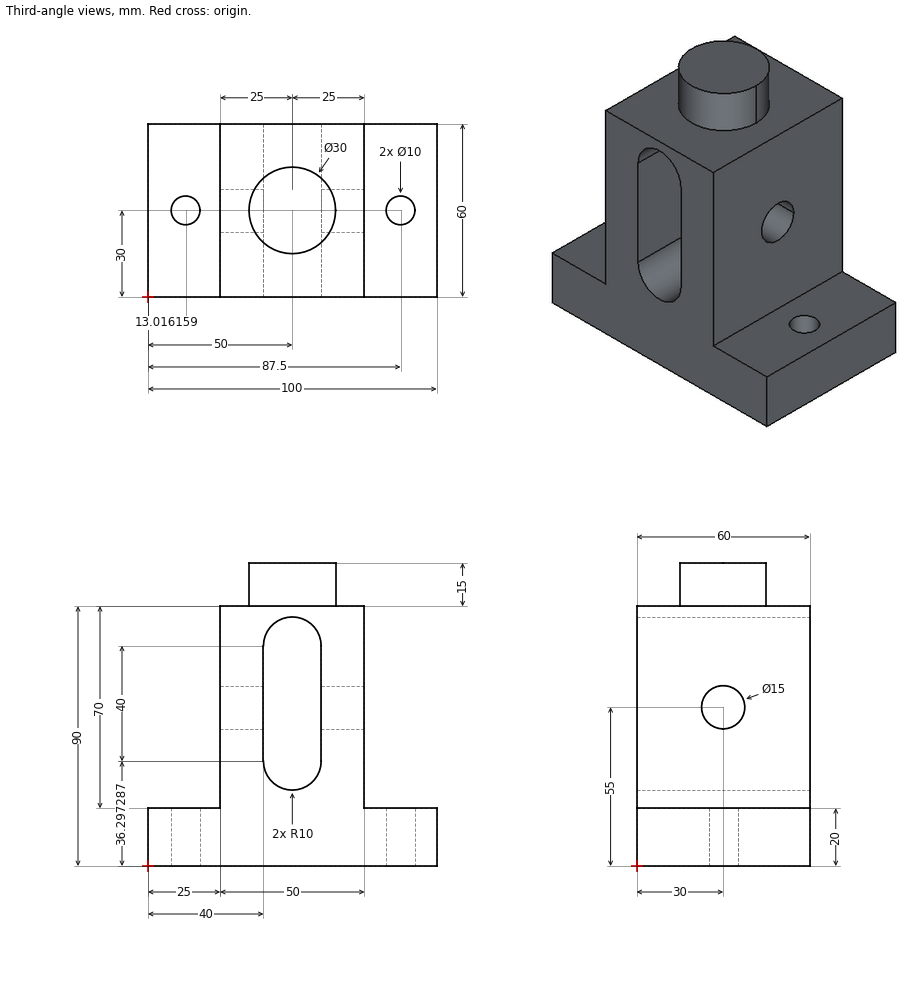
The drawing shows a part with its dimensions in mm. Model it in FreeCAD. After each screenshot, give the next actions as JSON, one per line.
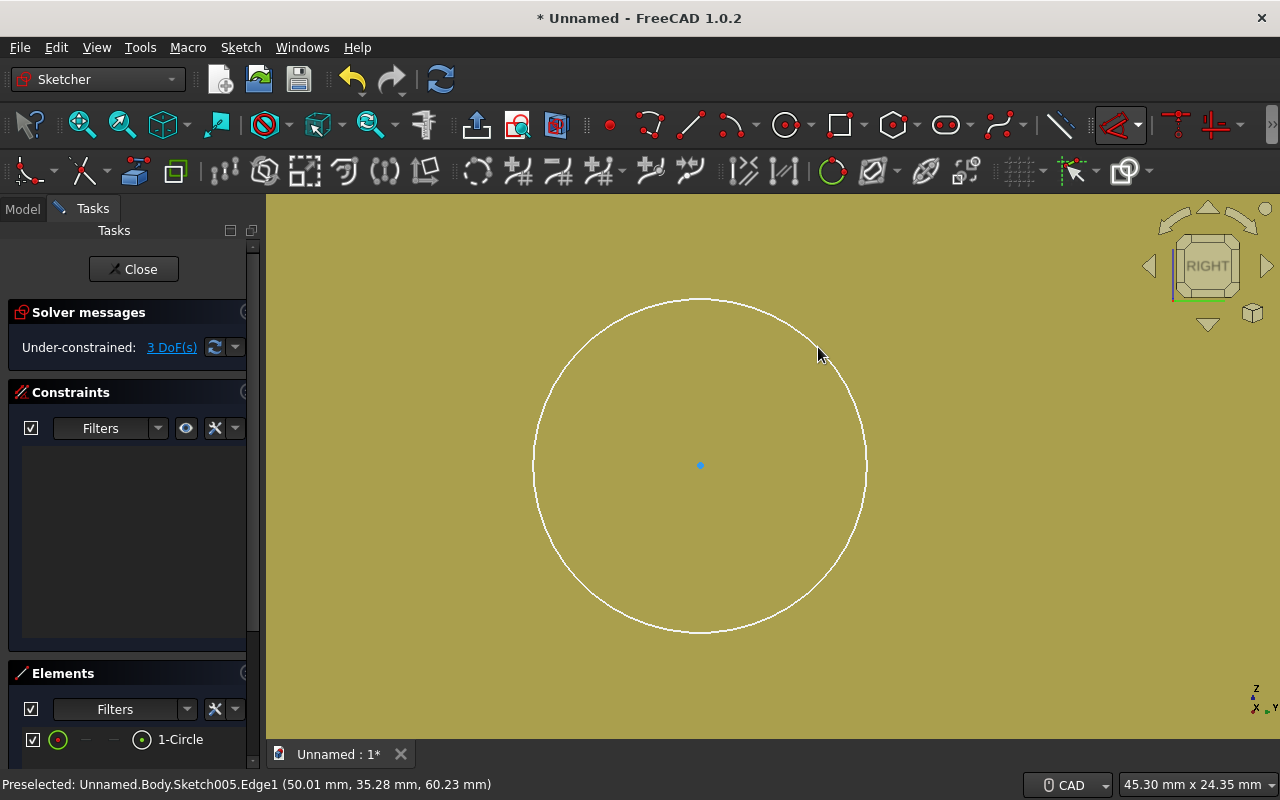
{"action": "left_click", "coordinate": [818, 348]}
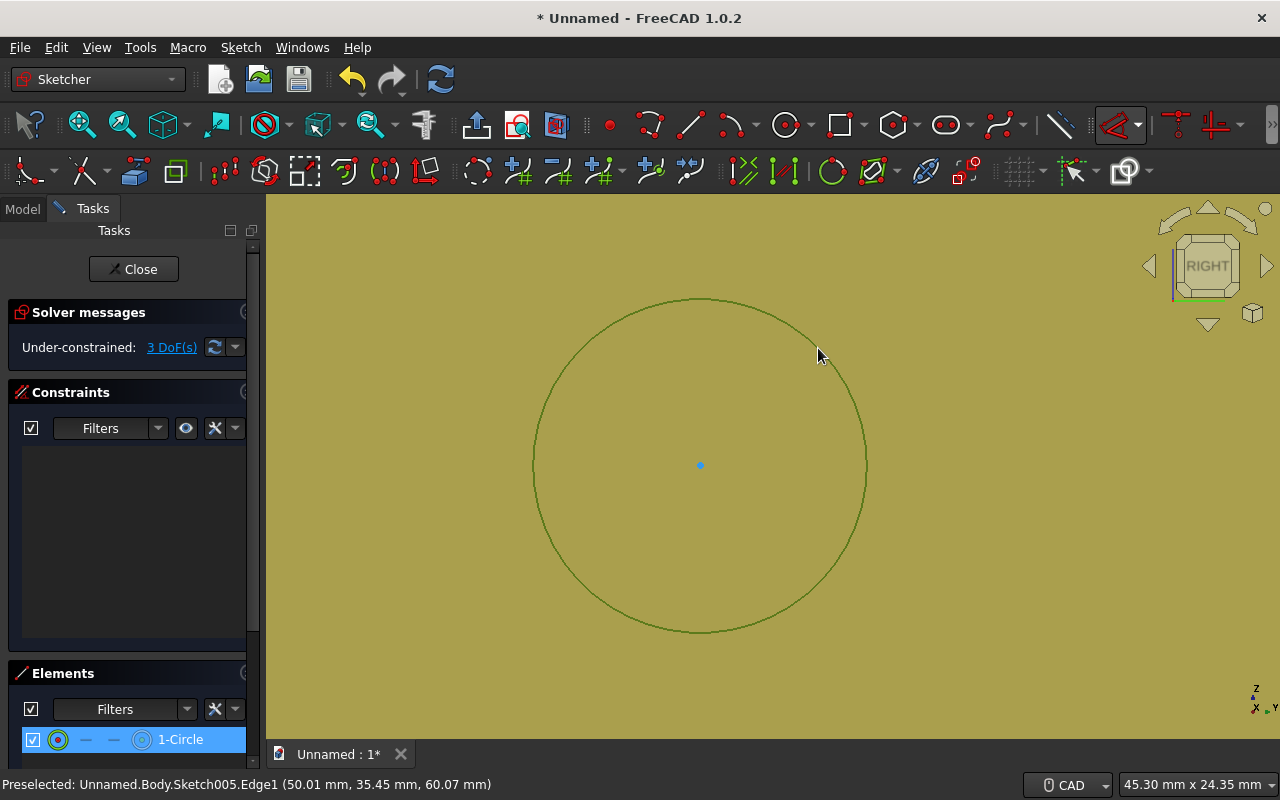
{"action": "key", "text": "k o"}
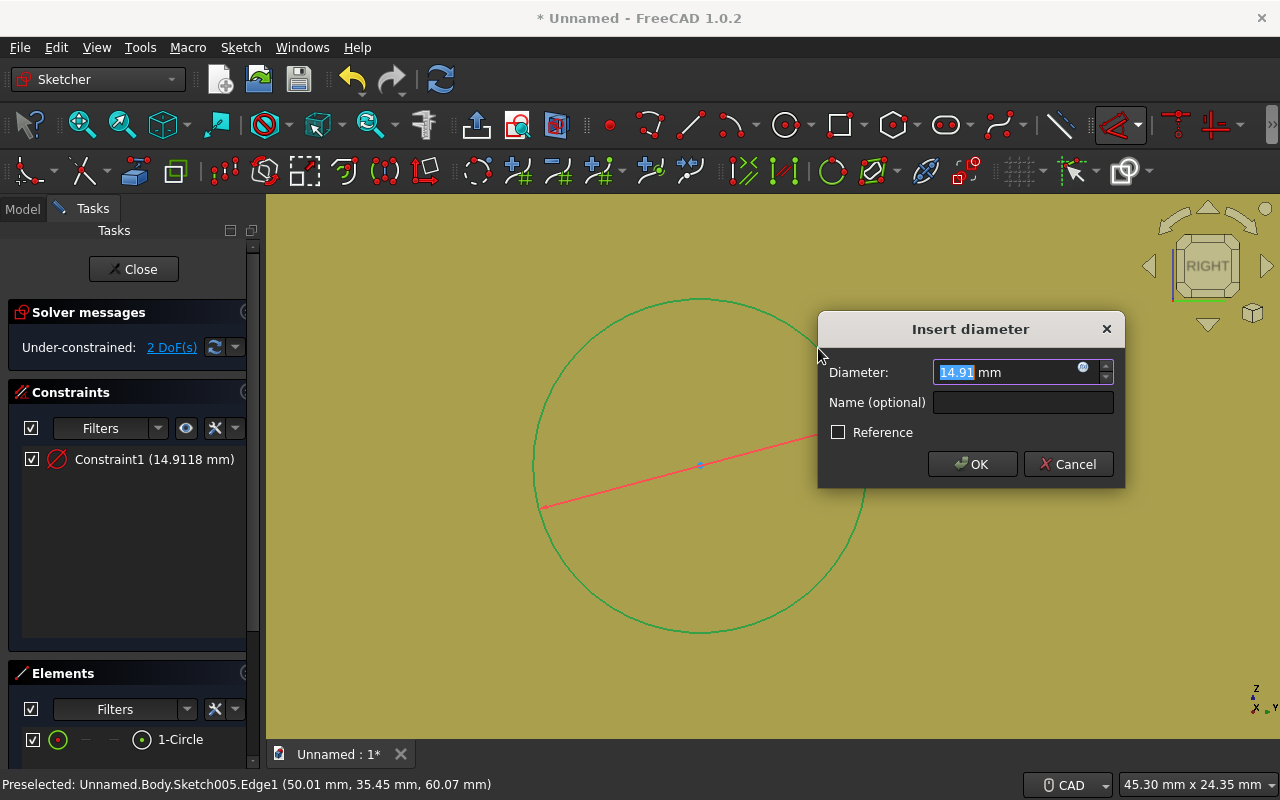
{"action": "type", "text": "15"}
{"action": "key", "text": "Return"}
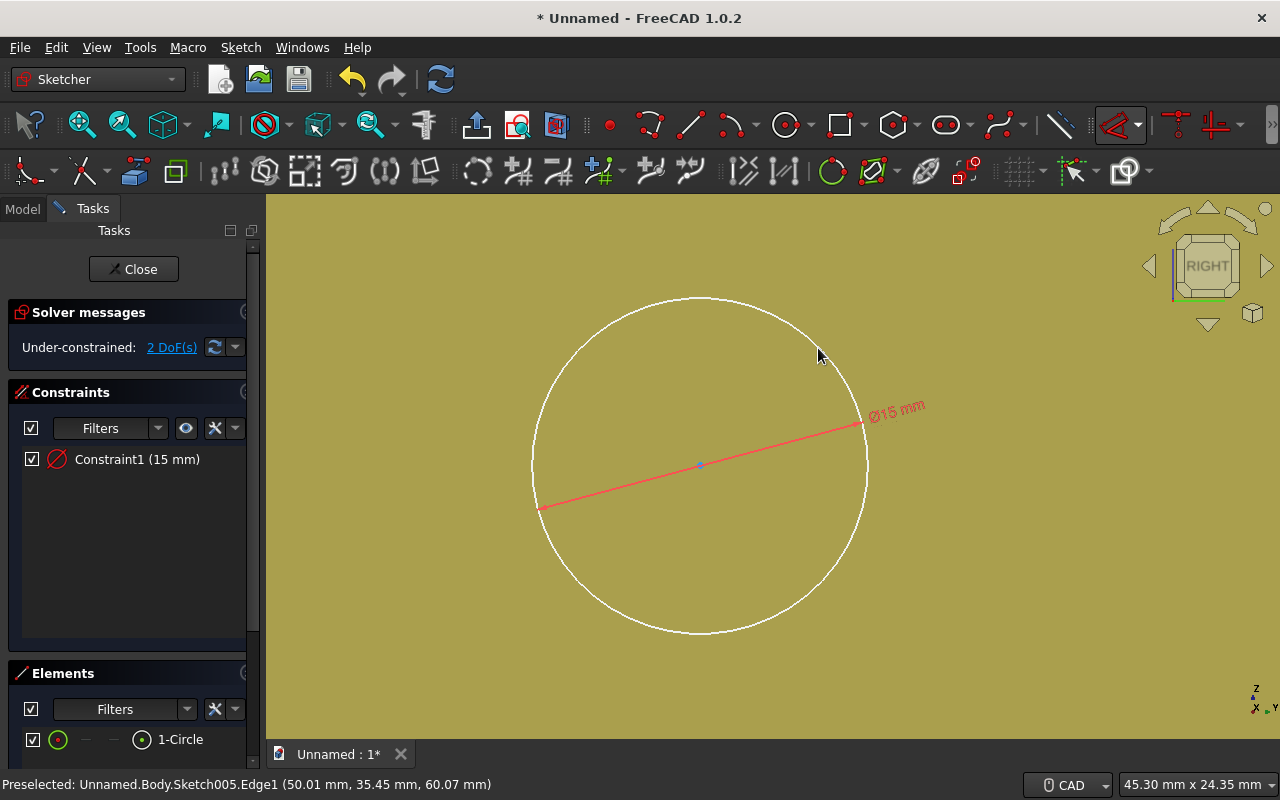
{"action": "left_click", "coordinate": [700, 466]}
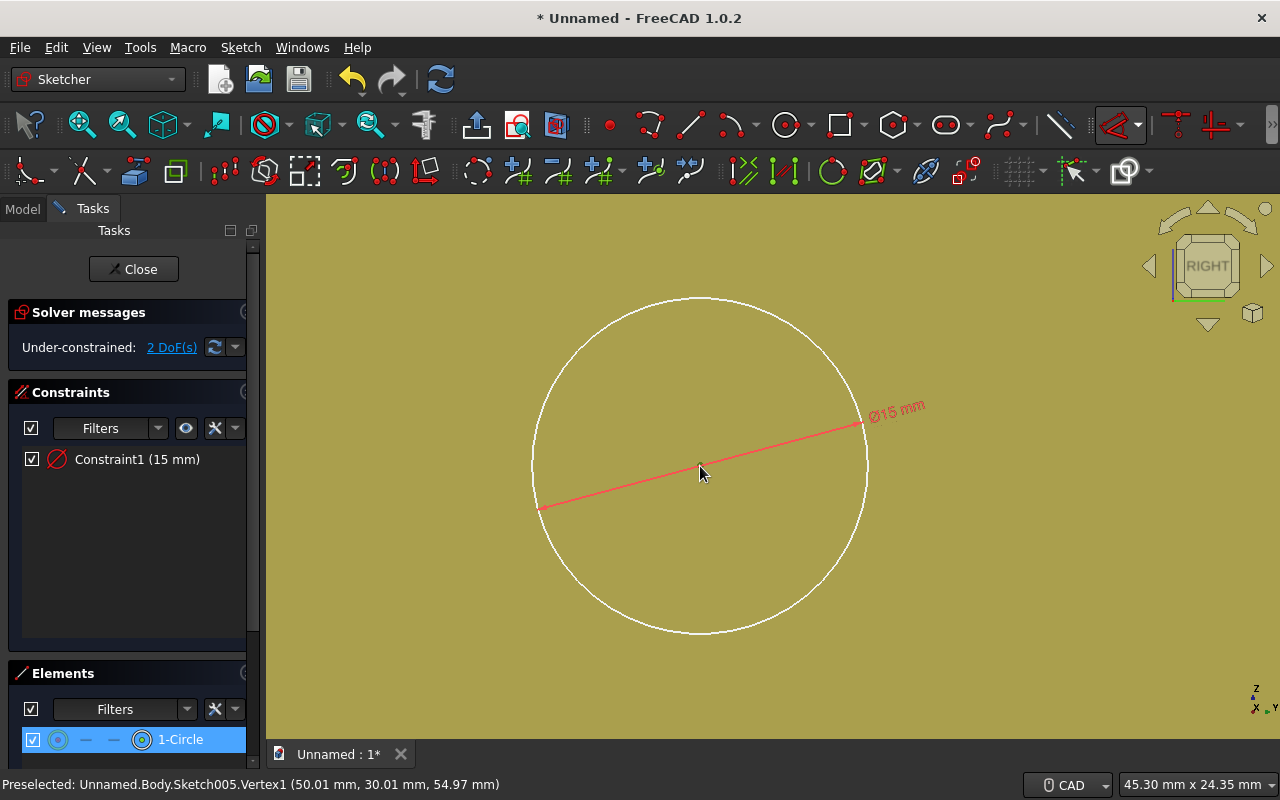
{"action": "key", "text": "l"}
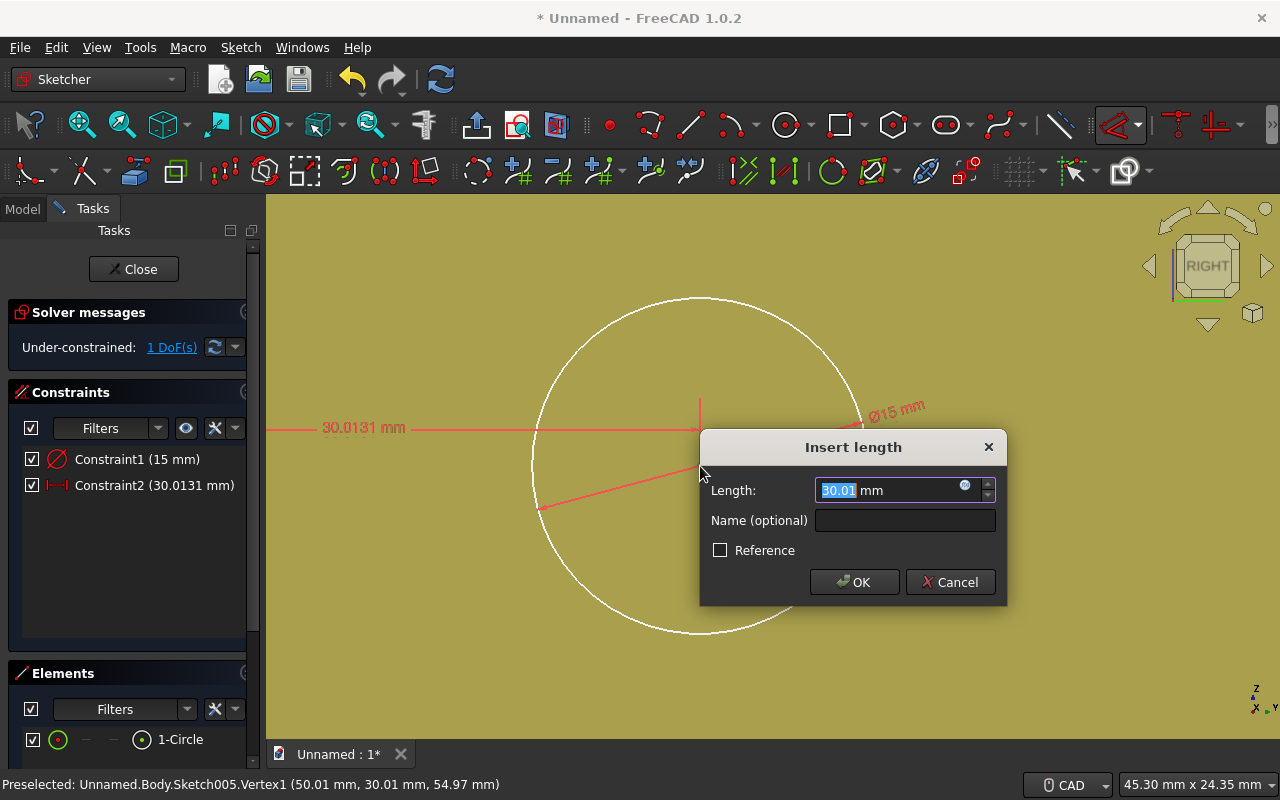
{"action": "type", "text": "30"}
{"action": "key", "text": "Return"}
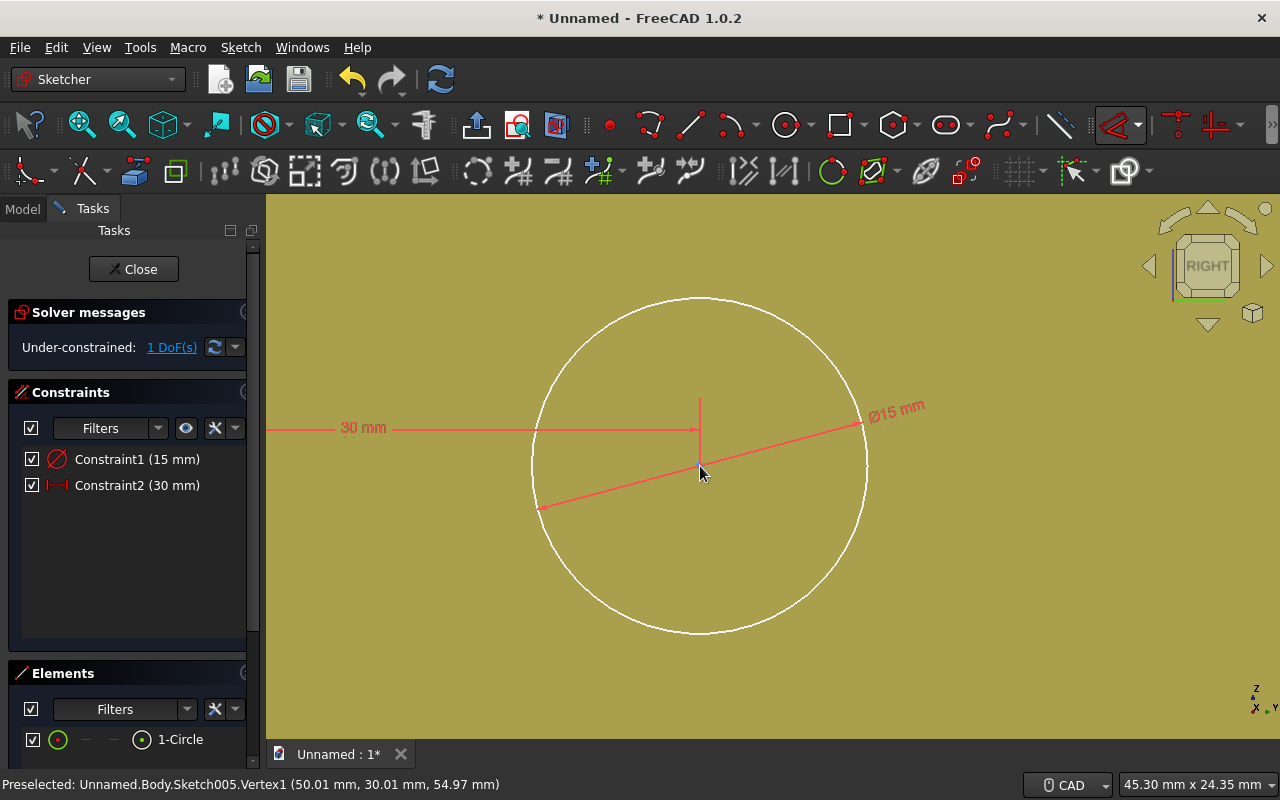
{"action": "left_click", "coordinate": [700, 466]}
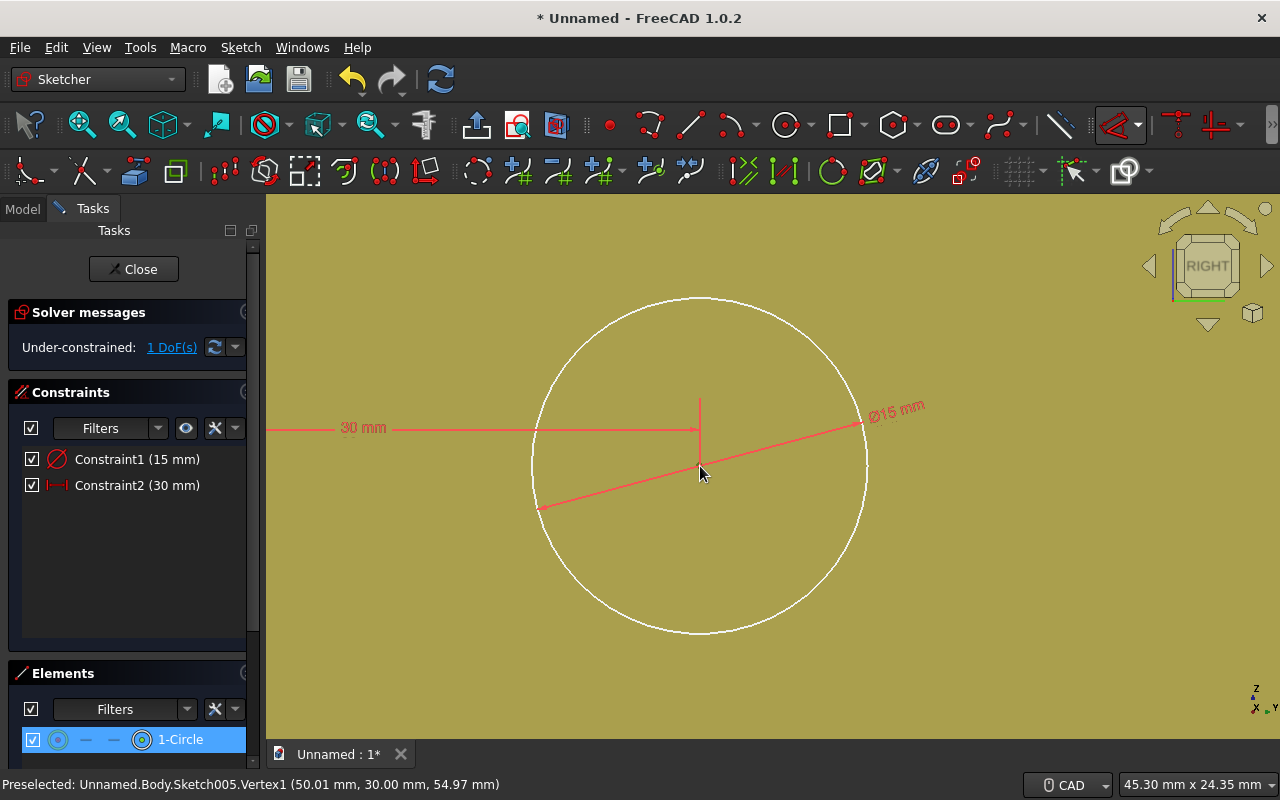
{"action": "key", "text": "i"}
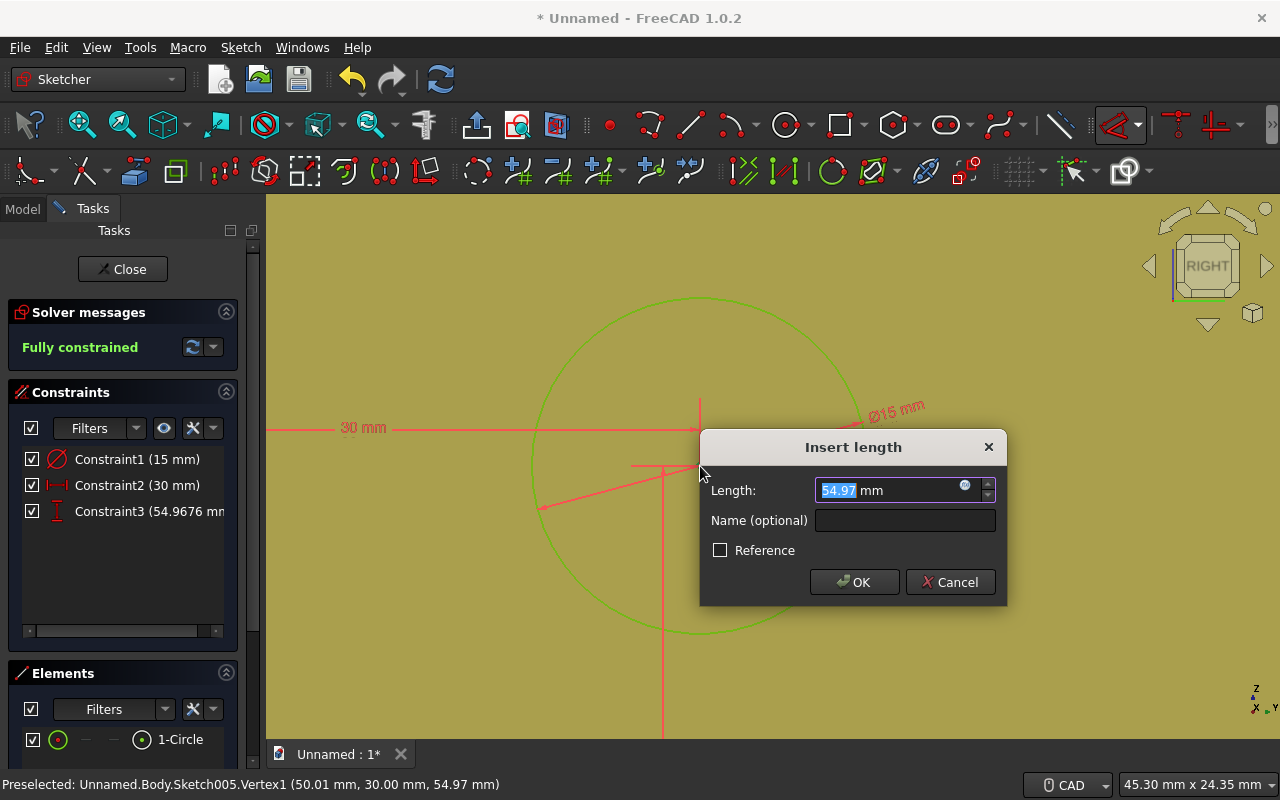
{"action": "type", "text": "55"}
{"action": "key", "text": "Return"}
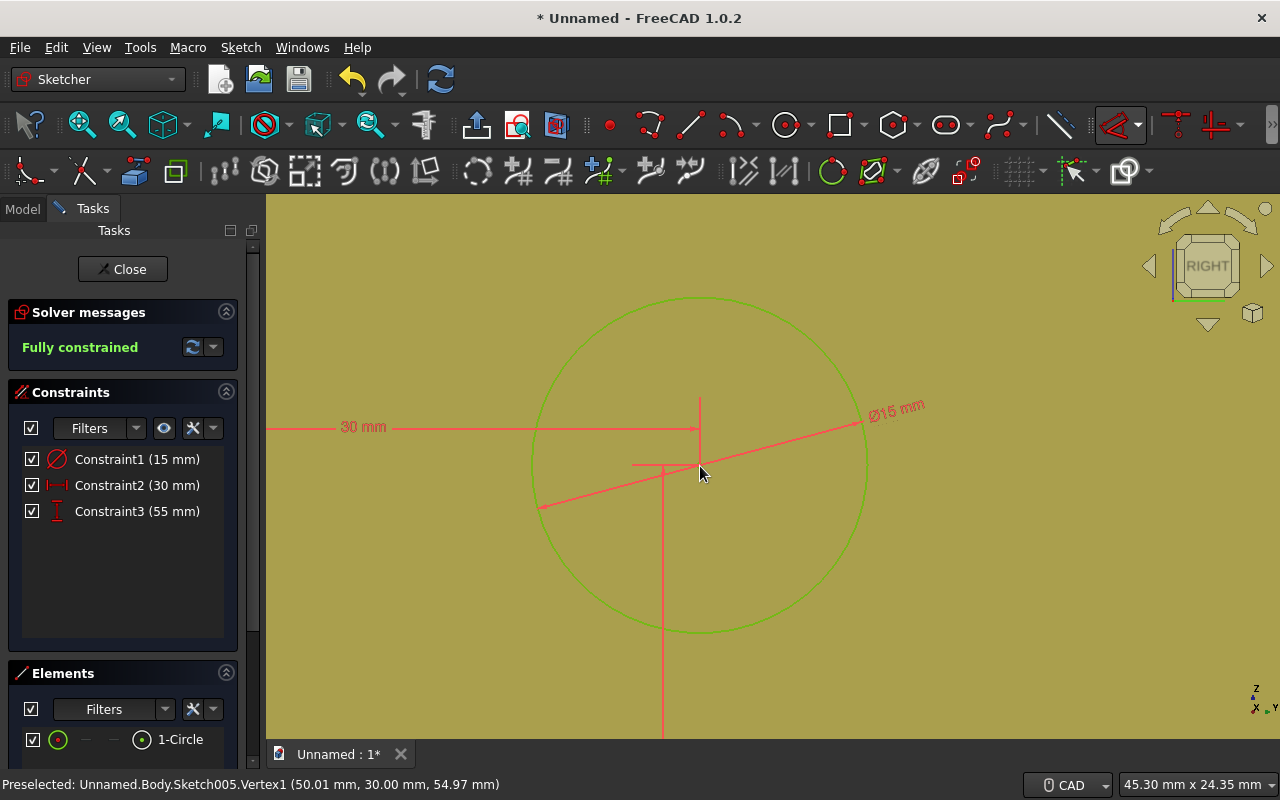
{"action": "left_click", "coordinate": [123, 269]}